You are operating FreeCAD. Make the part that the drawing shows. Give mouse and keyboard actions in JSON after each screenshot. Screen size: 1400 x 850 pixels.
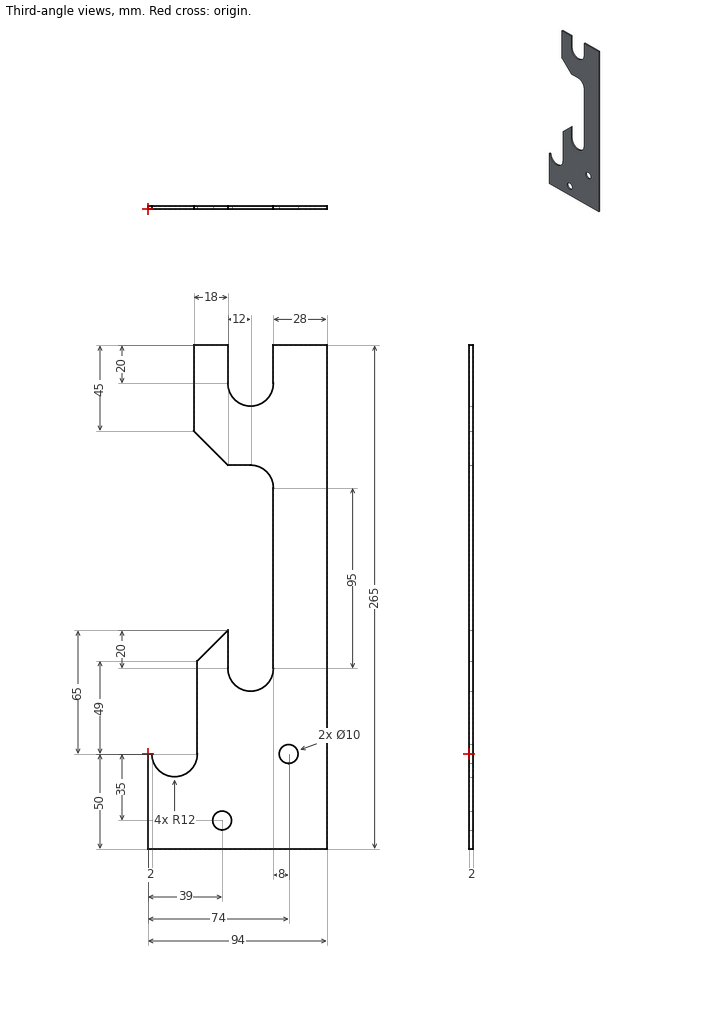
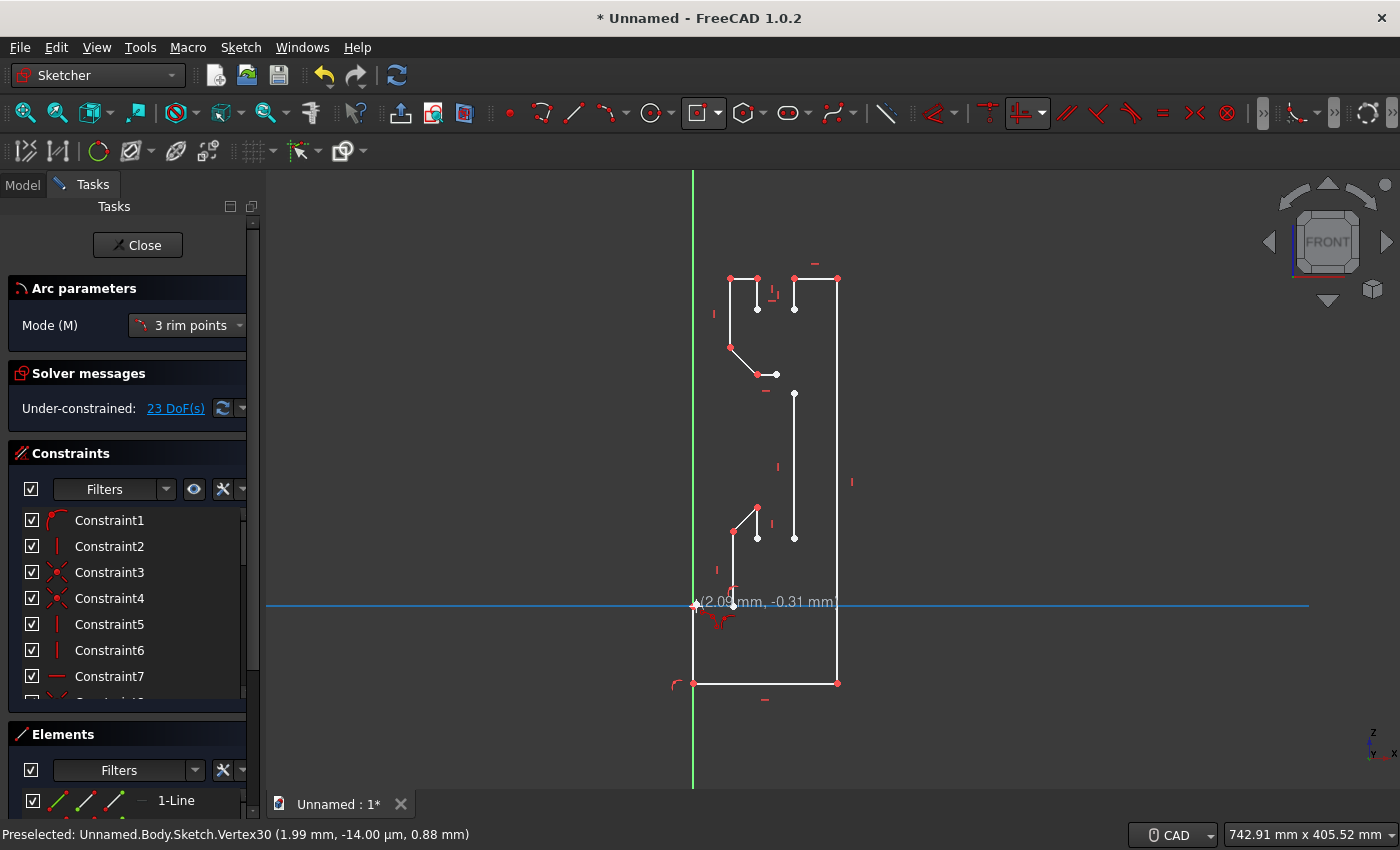
{"action": "left_click", "coordinate": [757, 539]}
{"action": "left_click", "coordinate": [794, 539]}
{"action": "left_click", "coordinate": [776, 556]}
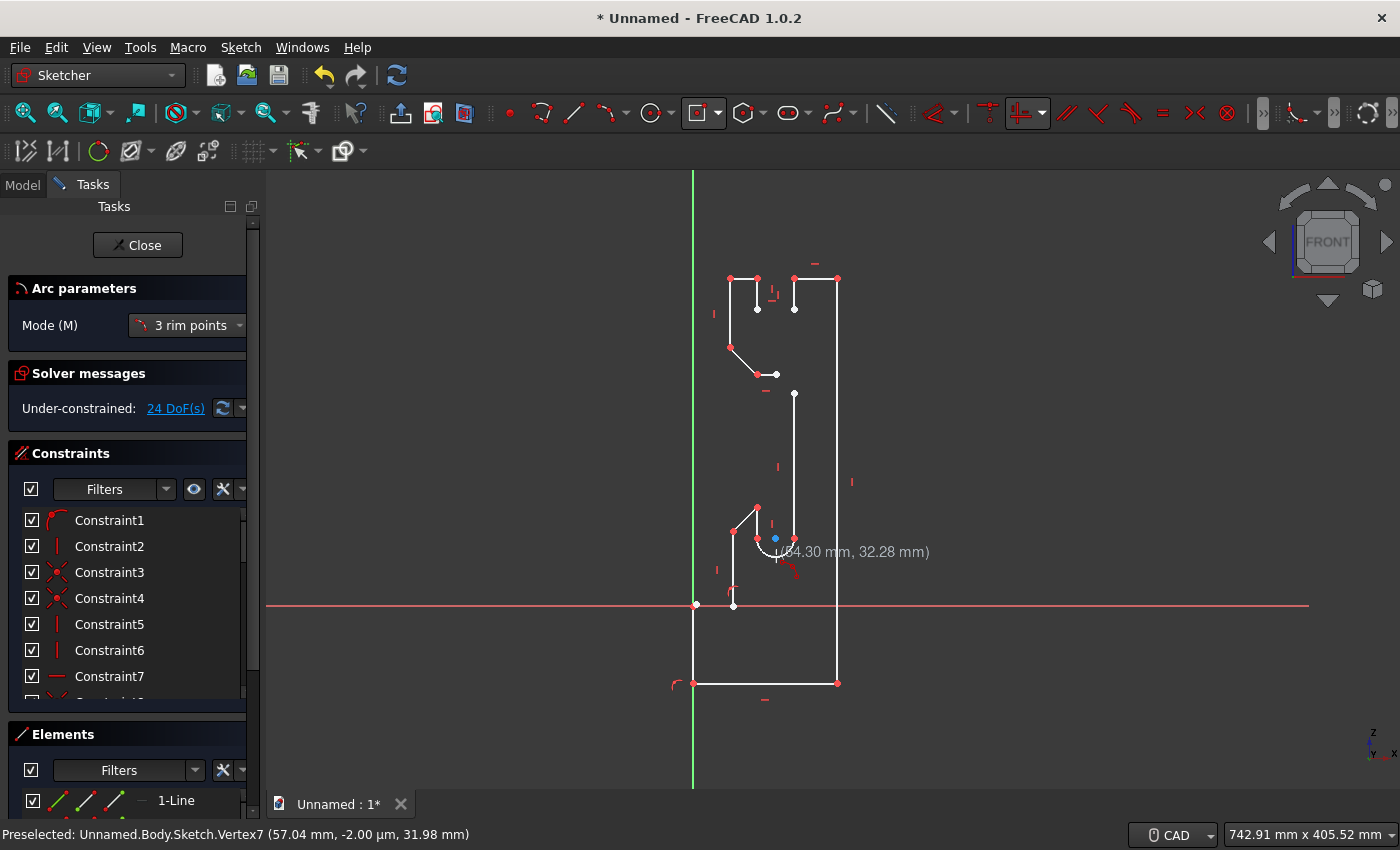
{"action": "left_click", "coordinate": [794, 394]}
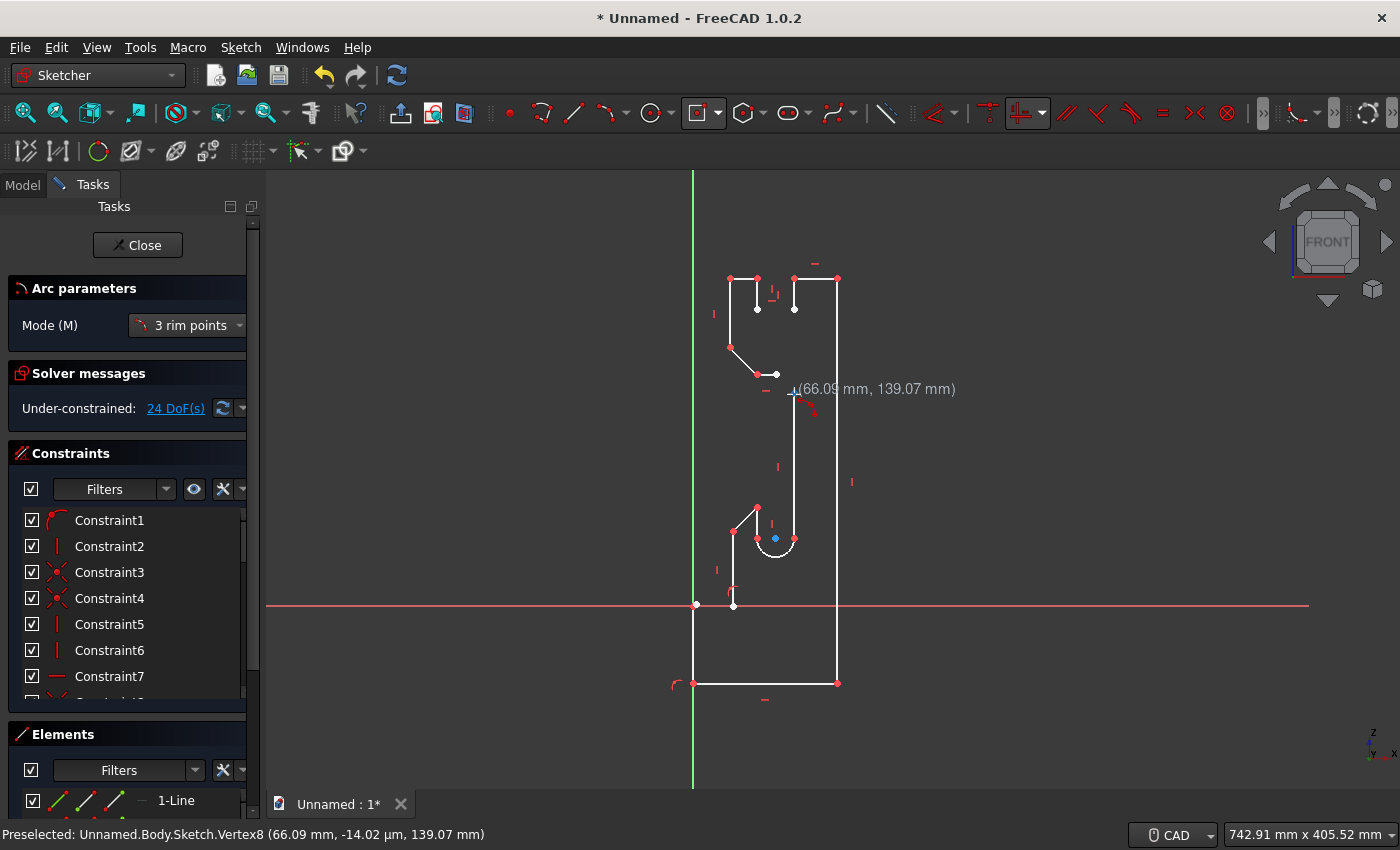
{"action": "scroll", "coordinate": [776, 374], "scroll_direction": "up", "scroll_amount": 3}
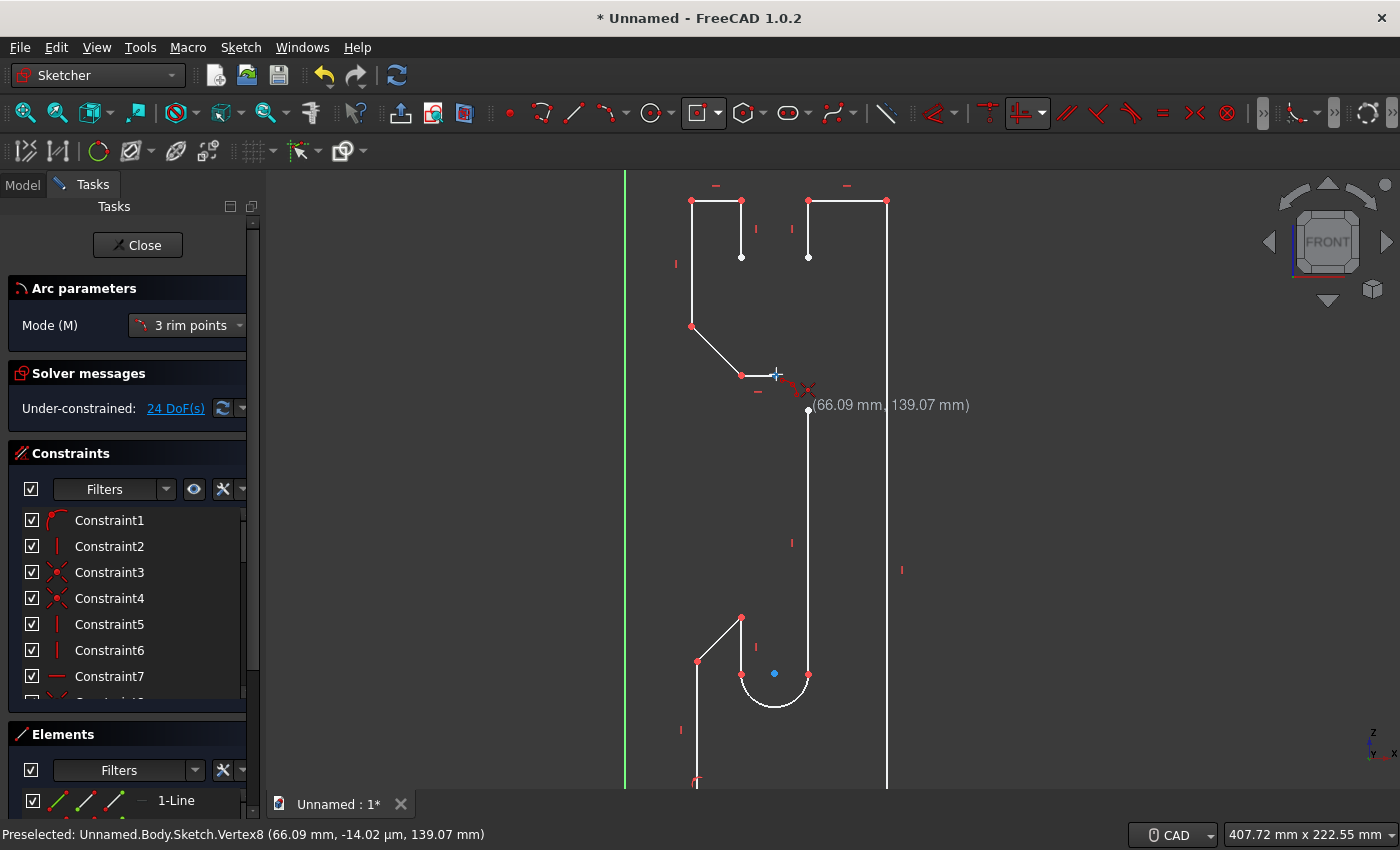
{"action": "left_click", "coordinate": [776, 376]}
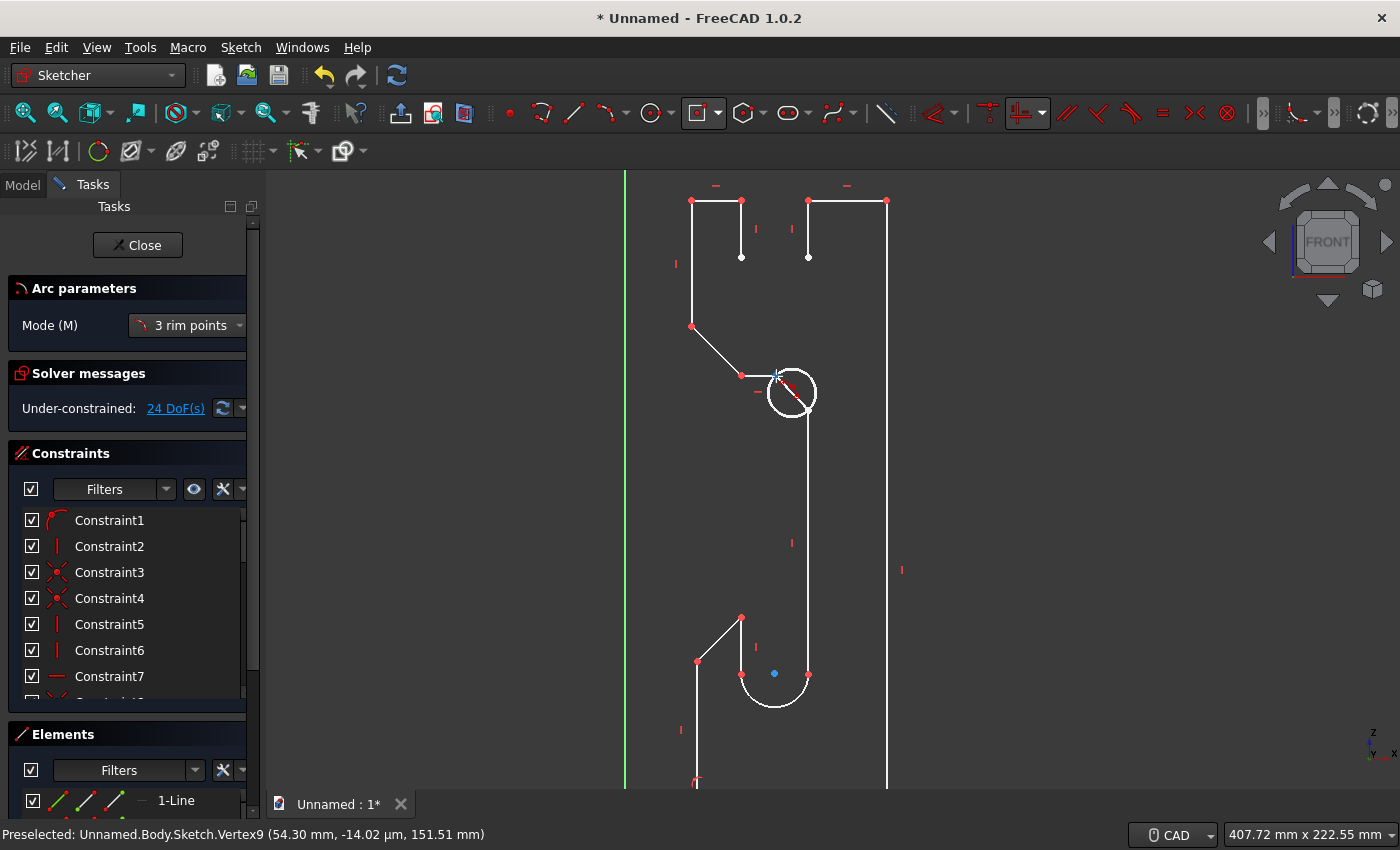
{"action": "scroll", "coordinate": [798, 384], "scroll_direction": "up", "scroll_amount": 3}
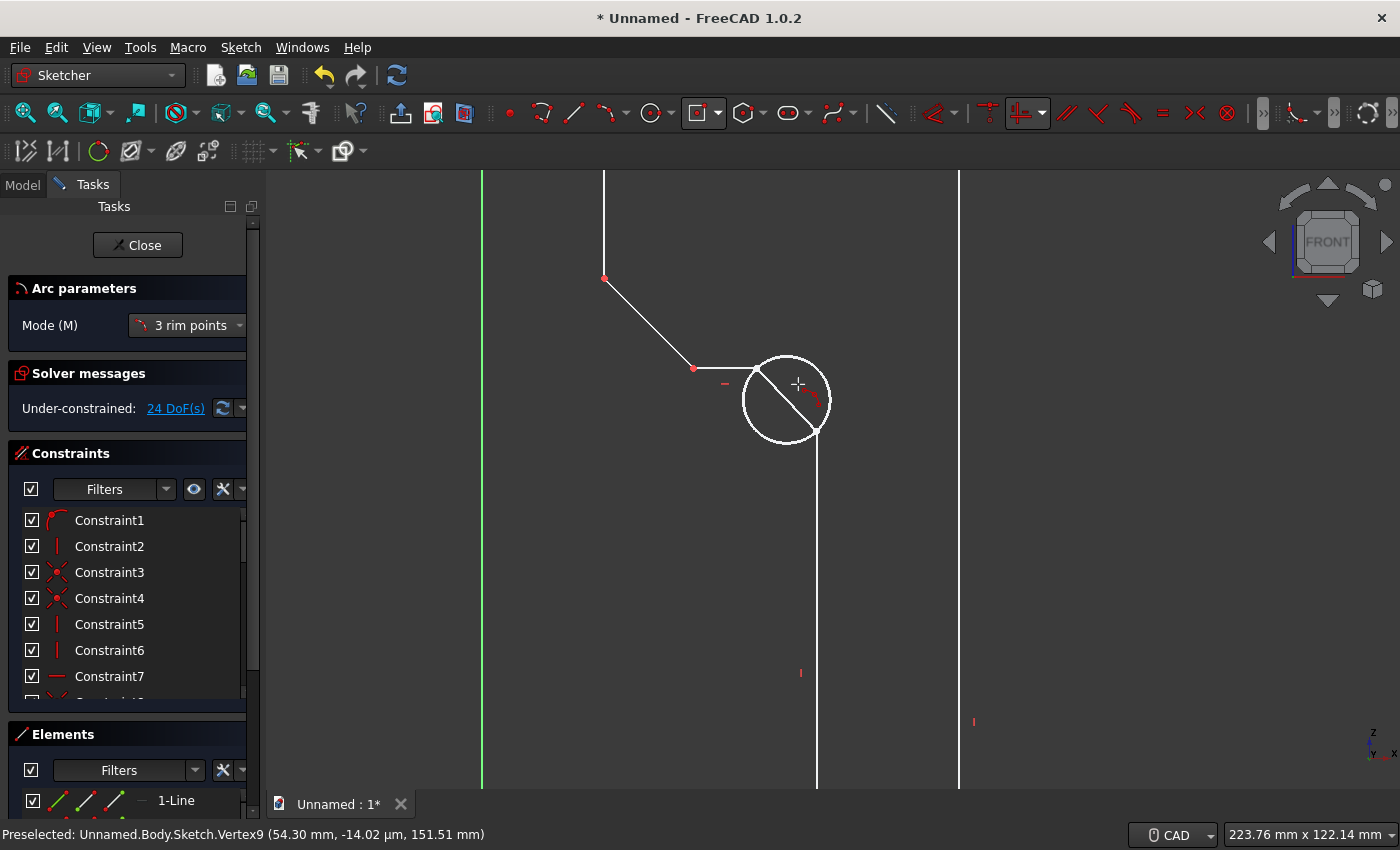
{"action": "left_click", "coordinate": [798, 384]}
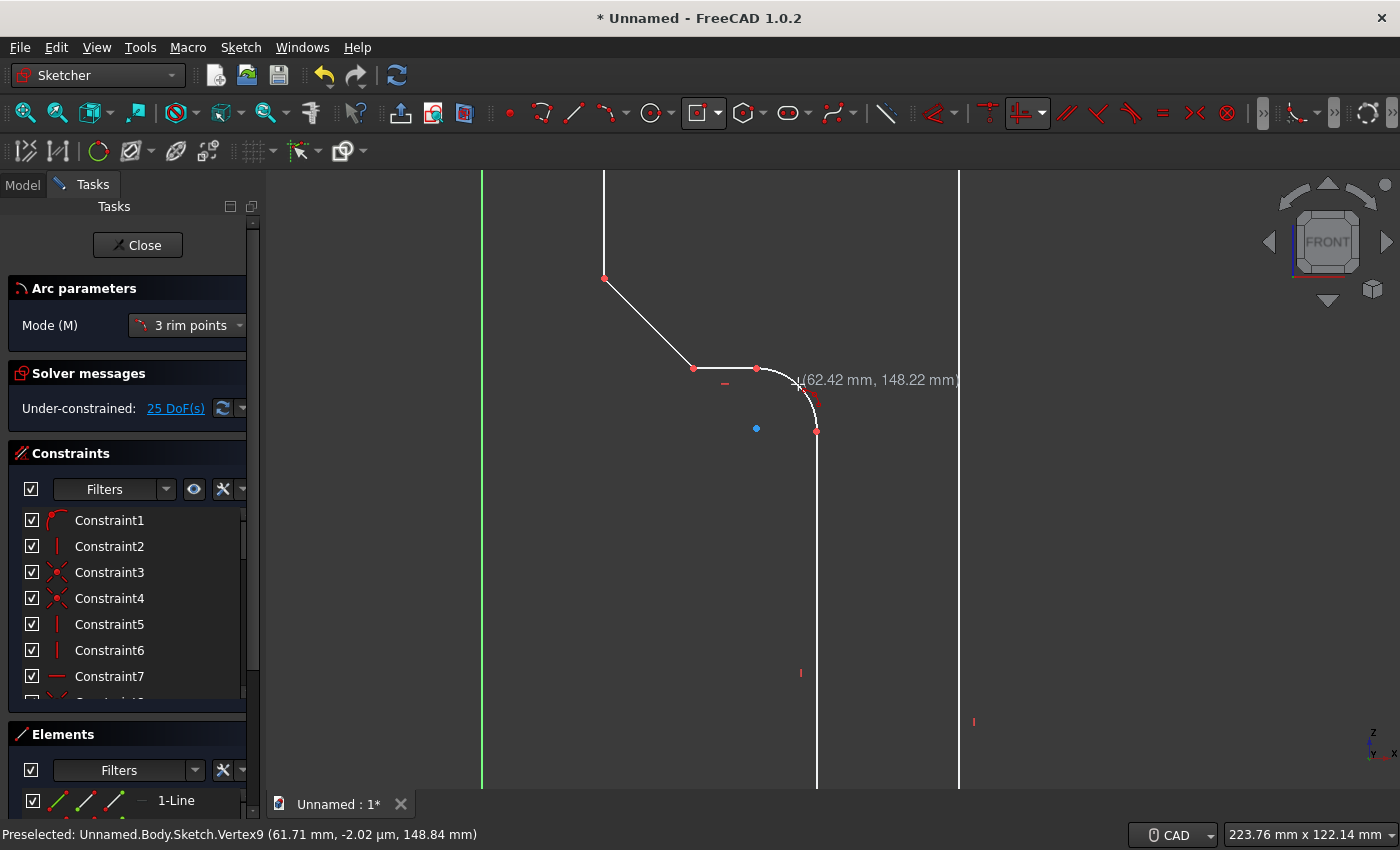
{"action": "scroll", "coordinate": [784, 377], "scroll_direction": "down", "scroll_amount": 6}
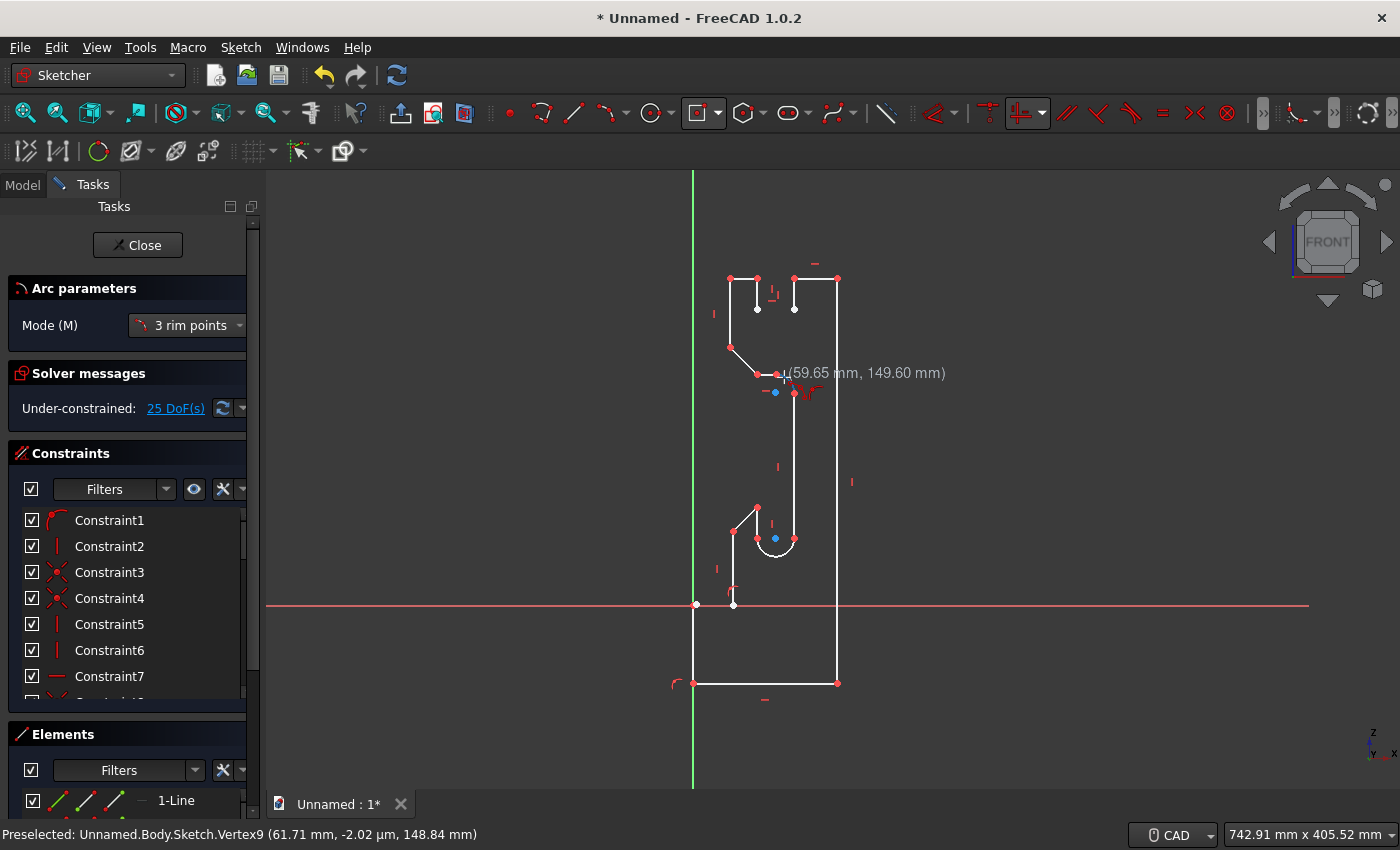
{"action": "left_click", "coordinate": [757, 310]}
{"action": "left_click", "coordinate": [794, 310]}
{"action": "left_click", "coordinate": [776, 327]}